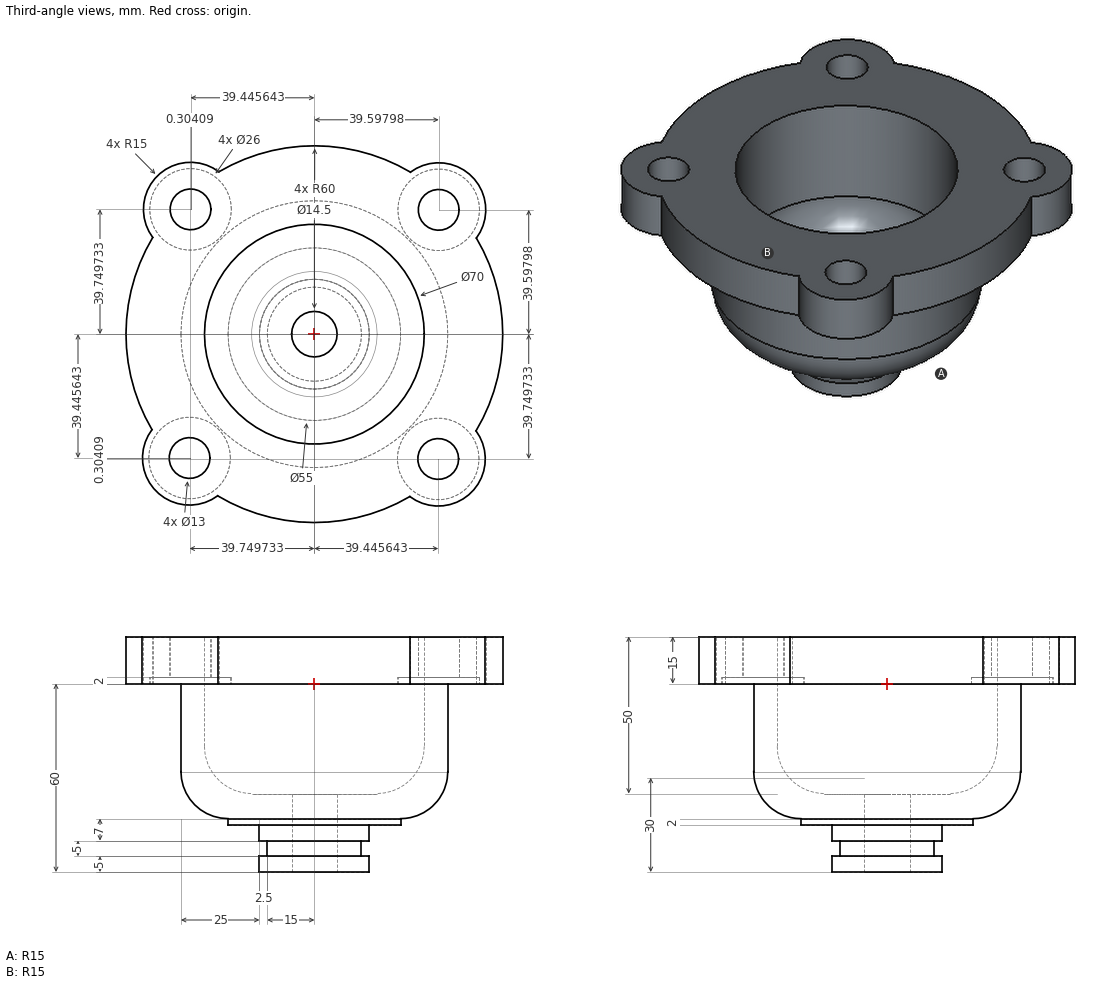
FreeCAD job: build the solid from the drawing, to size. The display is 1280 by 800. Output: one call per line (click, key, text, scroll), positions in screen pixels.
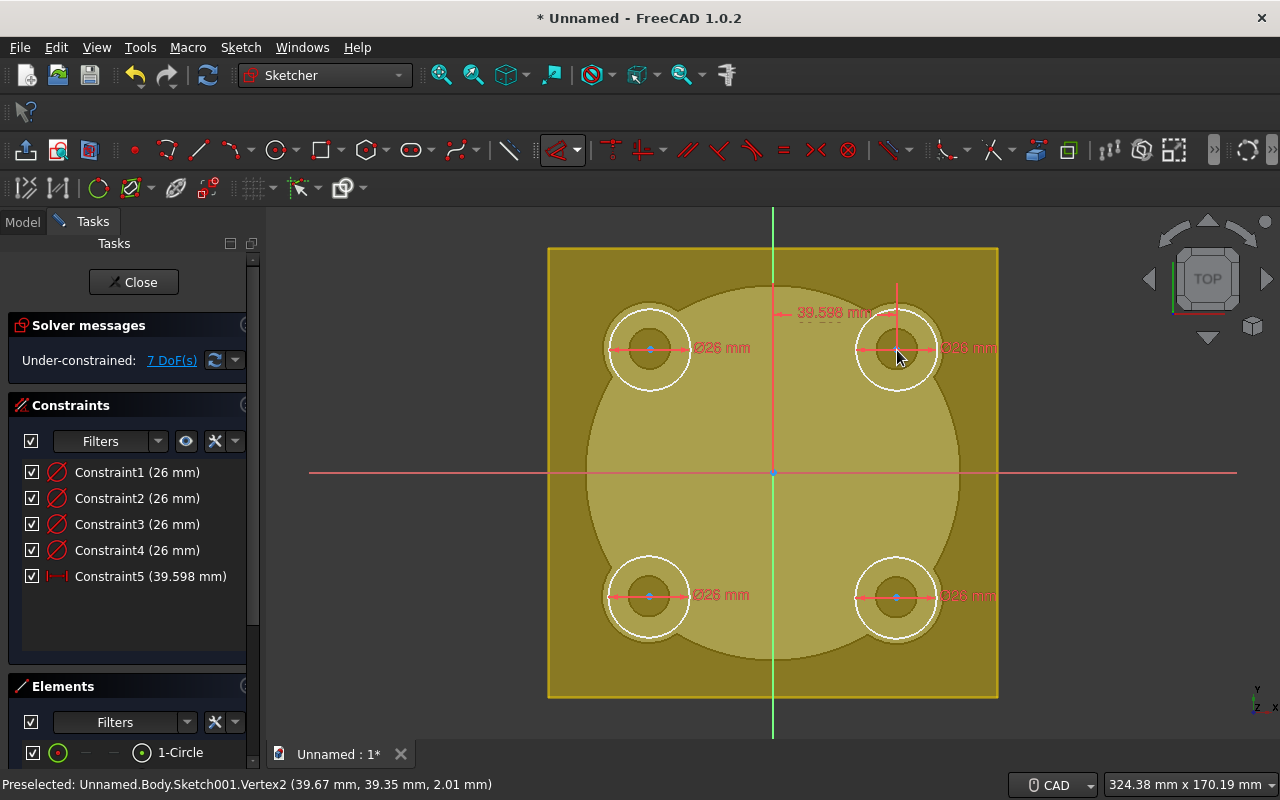
click(897, 350)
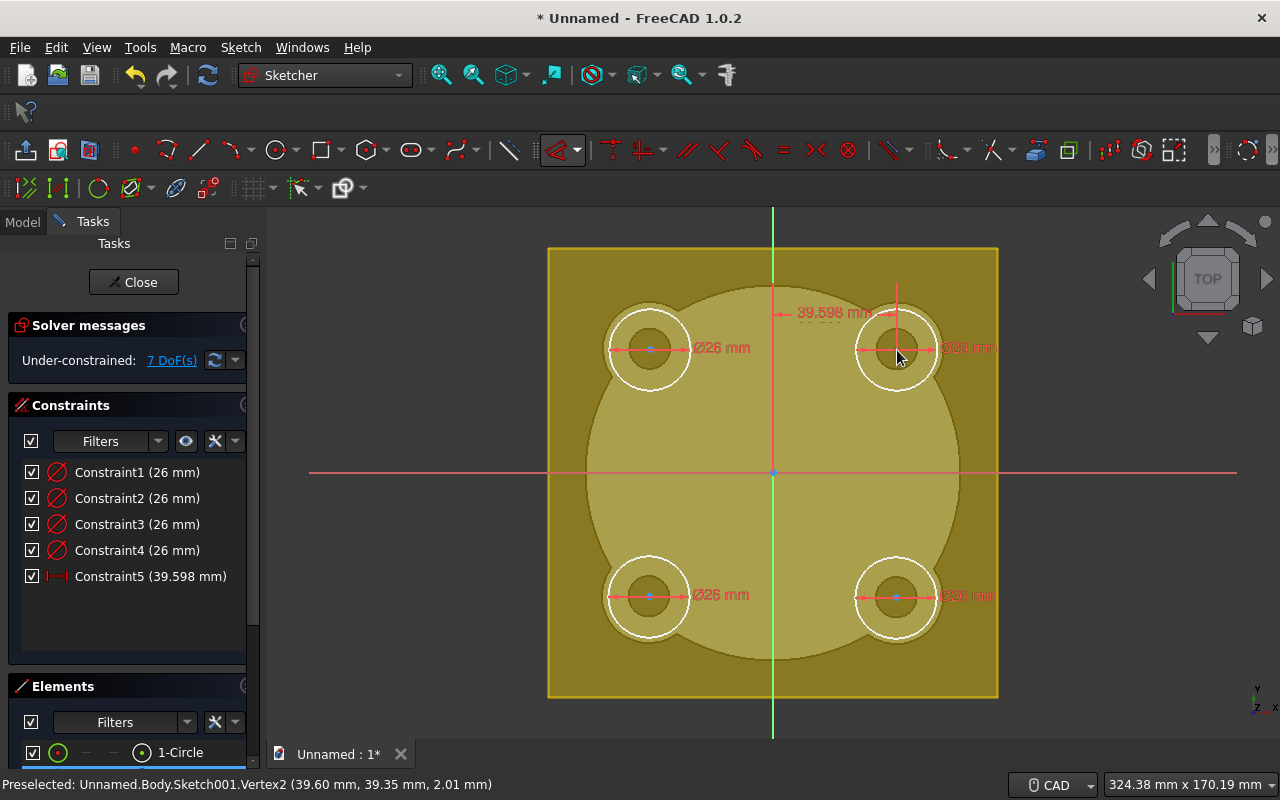
click(580, 150)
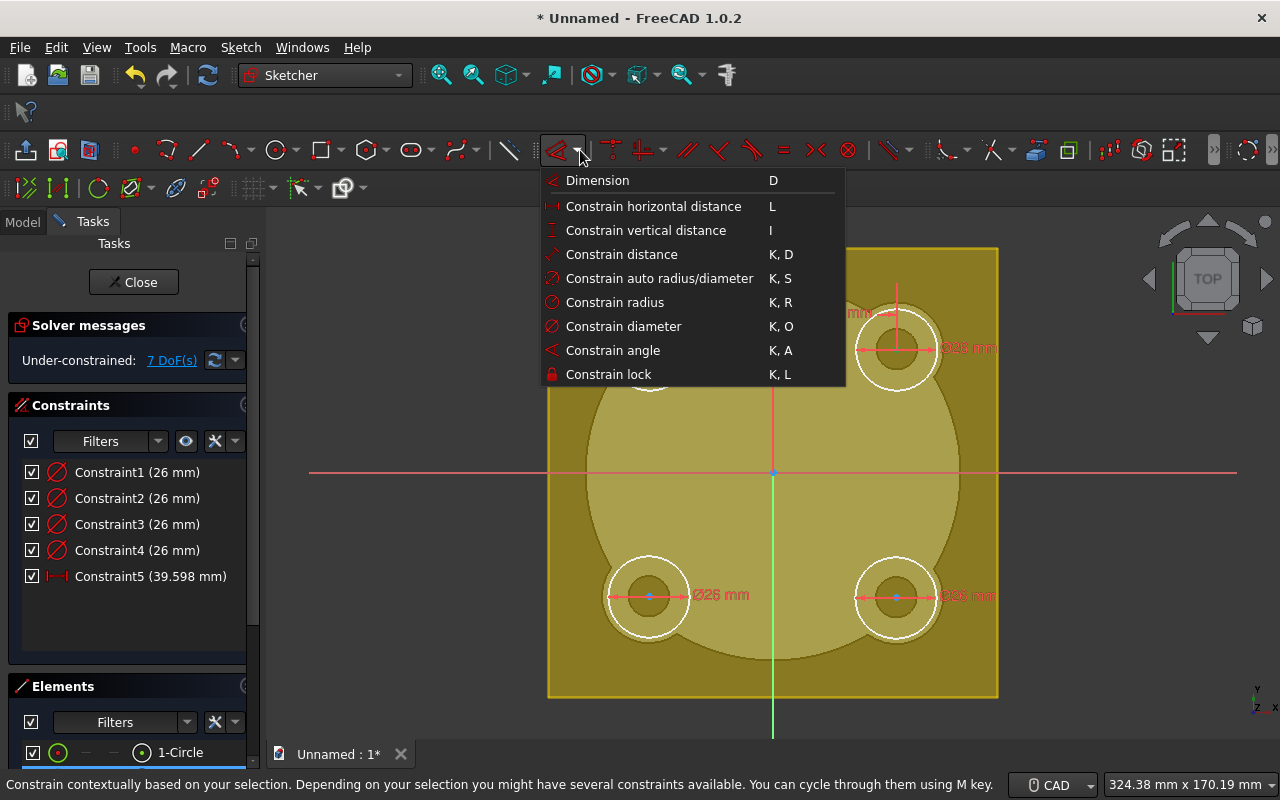
click(693, 230)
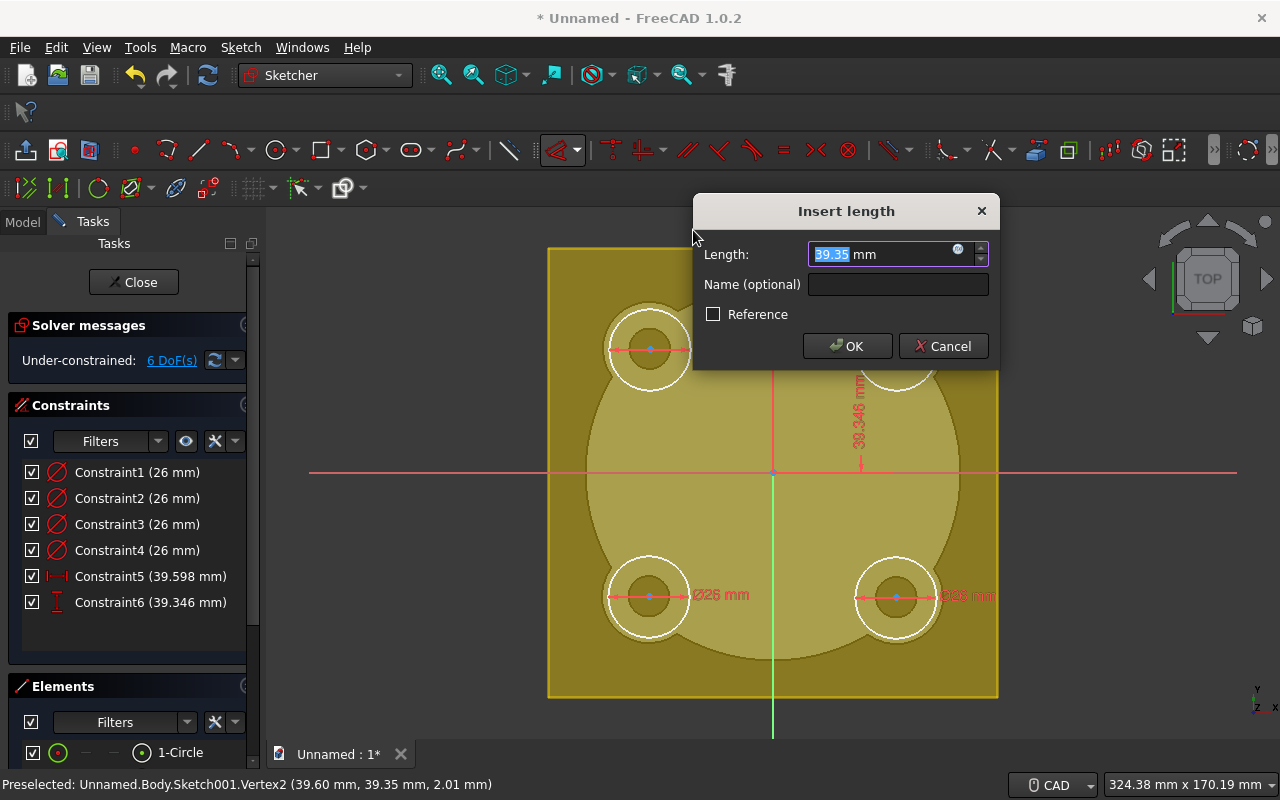
text(39.59798)
key(Return)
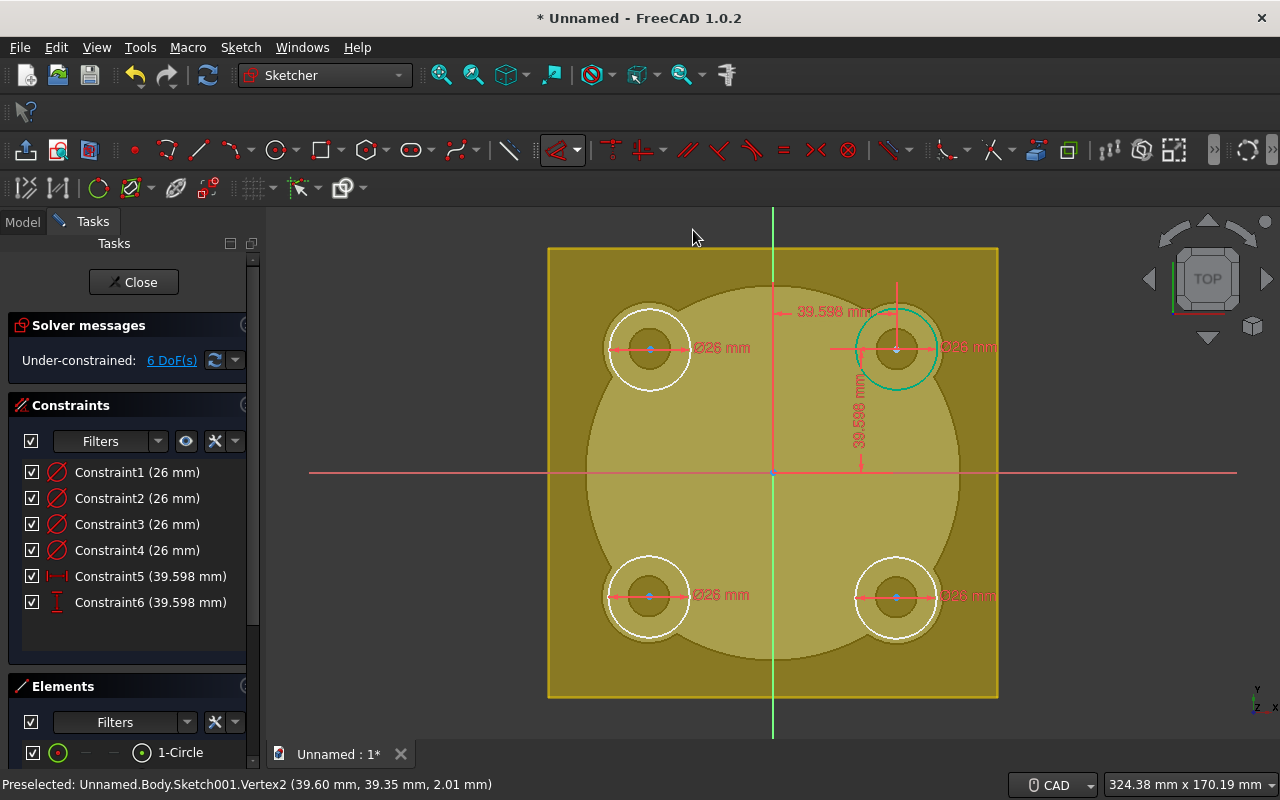
scroll(650, 350, up, 19)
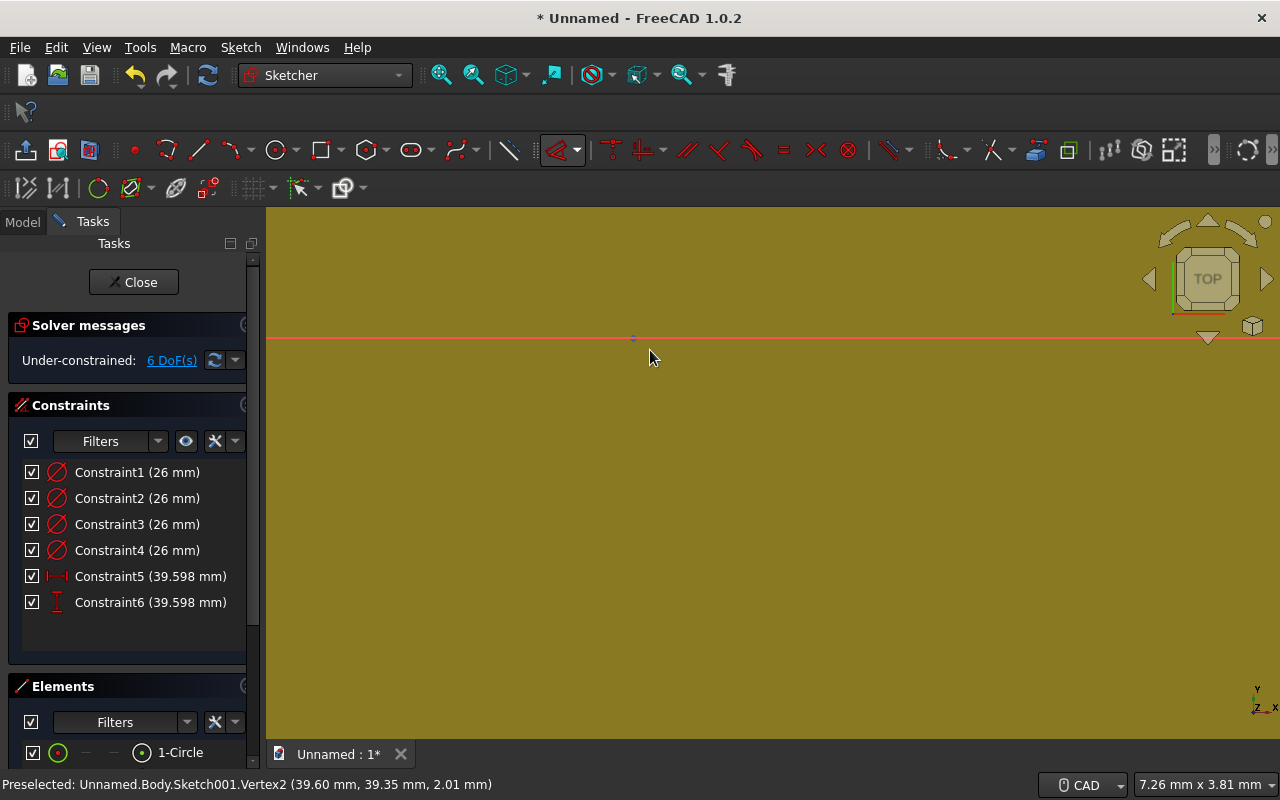
click(633, 338)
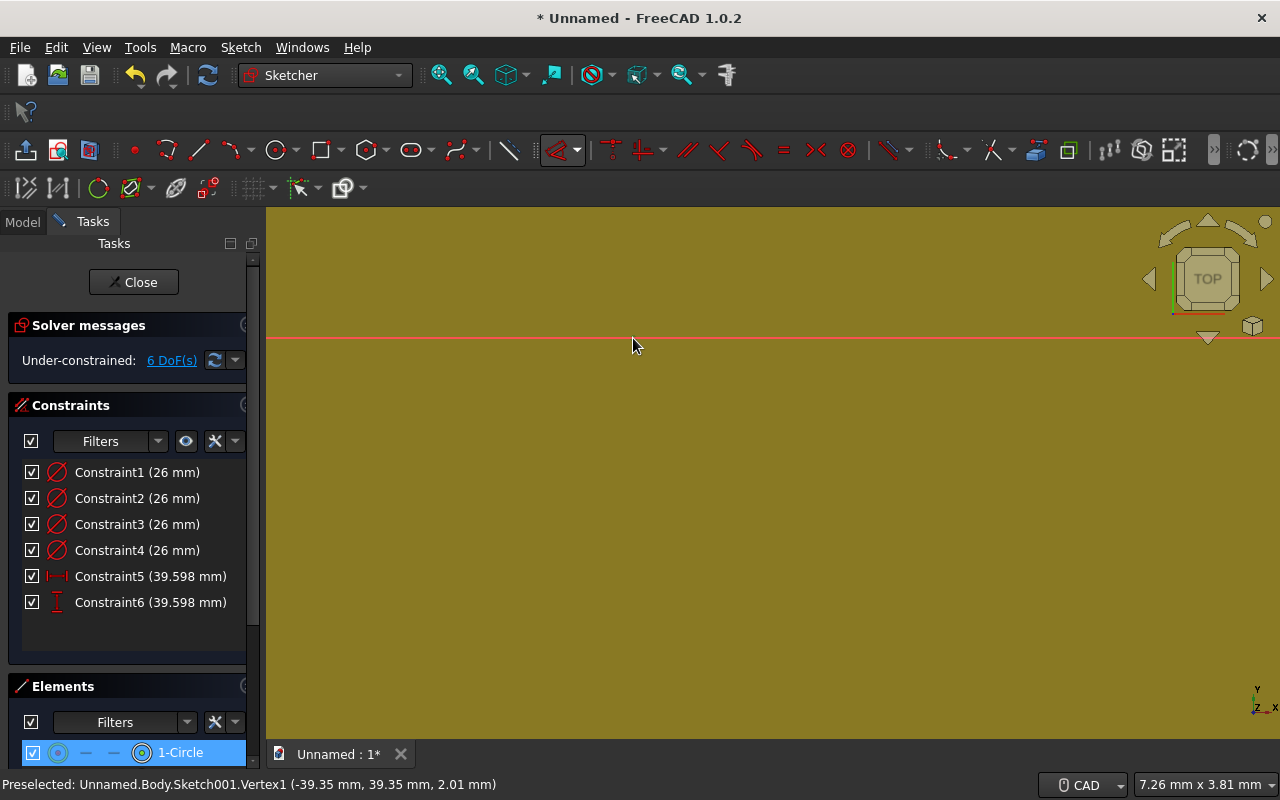
scroll(552, 322, down, 18)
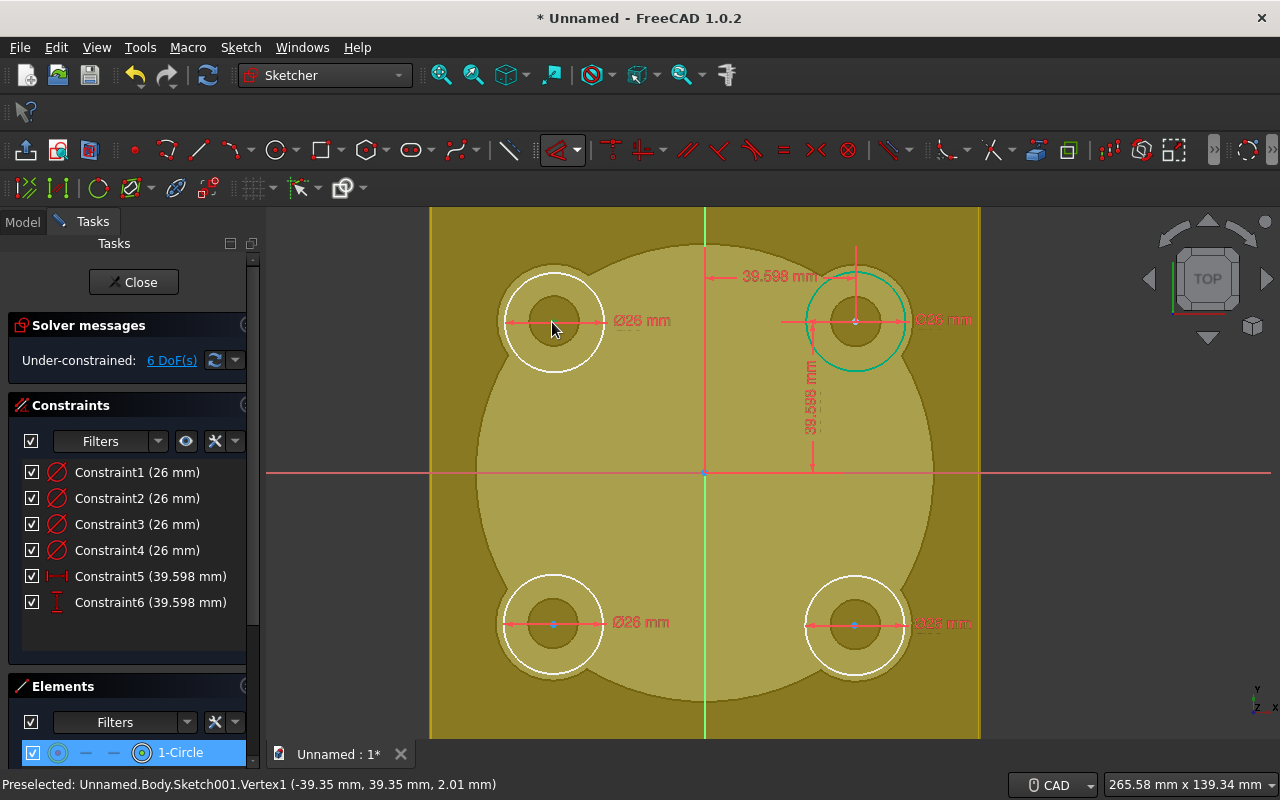
scroll(553, 624, up, 18)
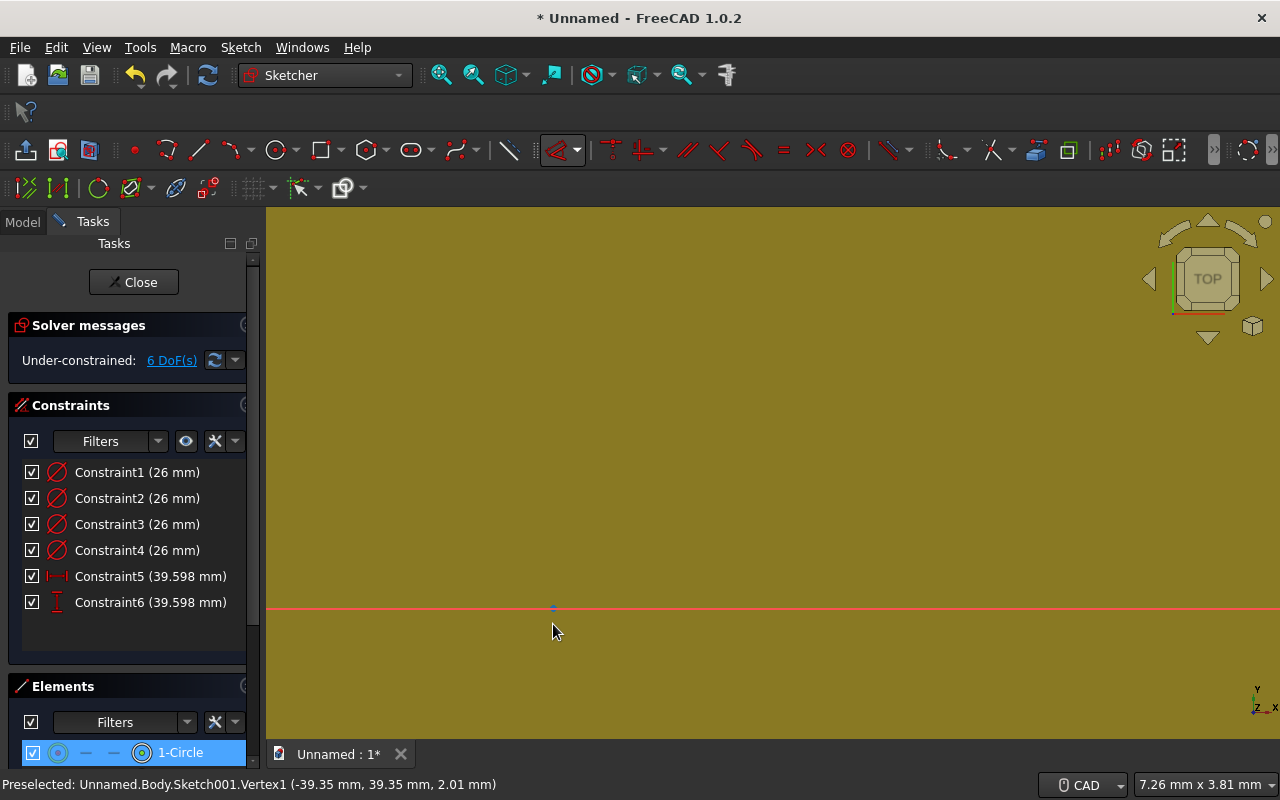
click(553, 609)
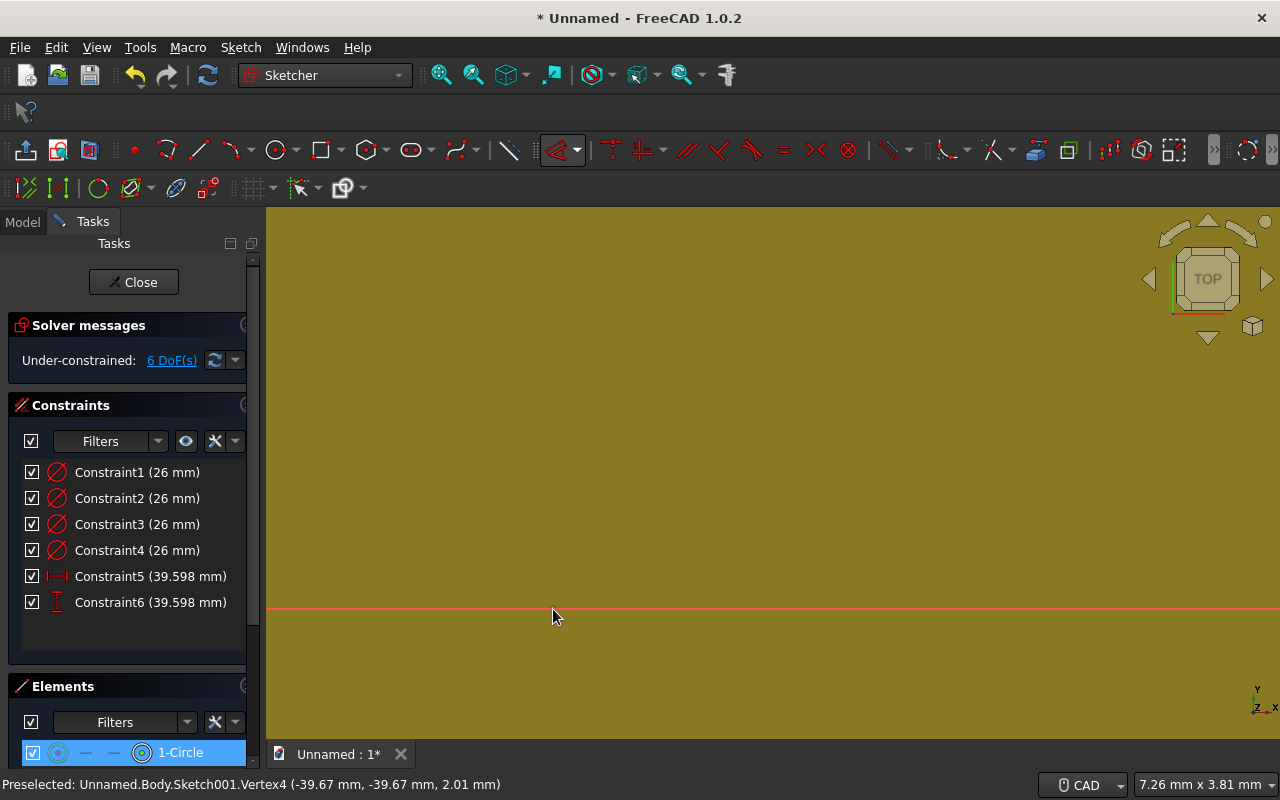
key(l)